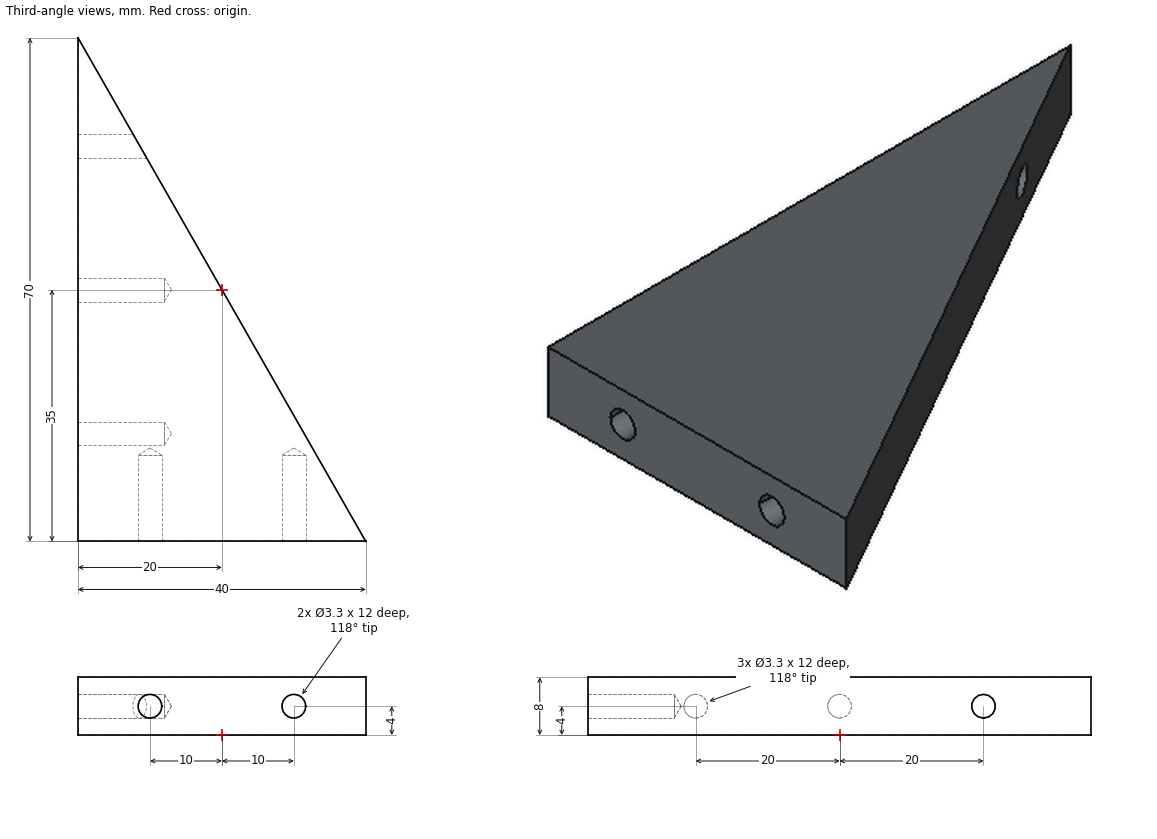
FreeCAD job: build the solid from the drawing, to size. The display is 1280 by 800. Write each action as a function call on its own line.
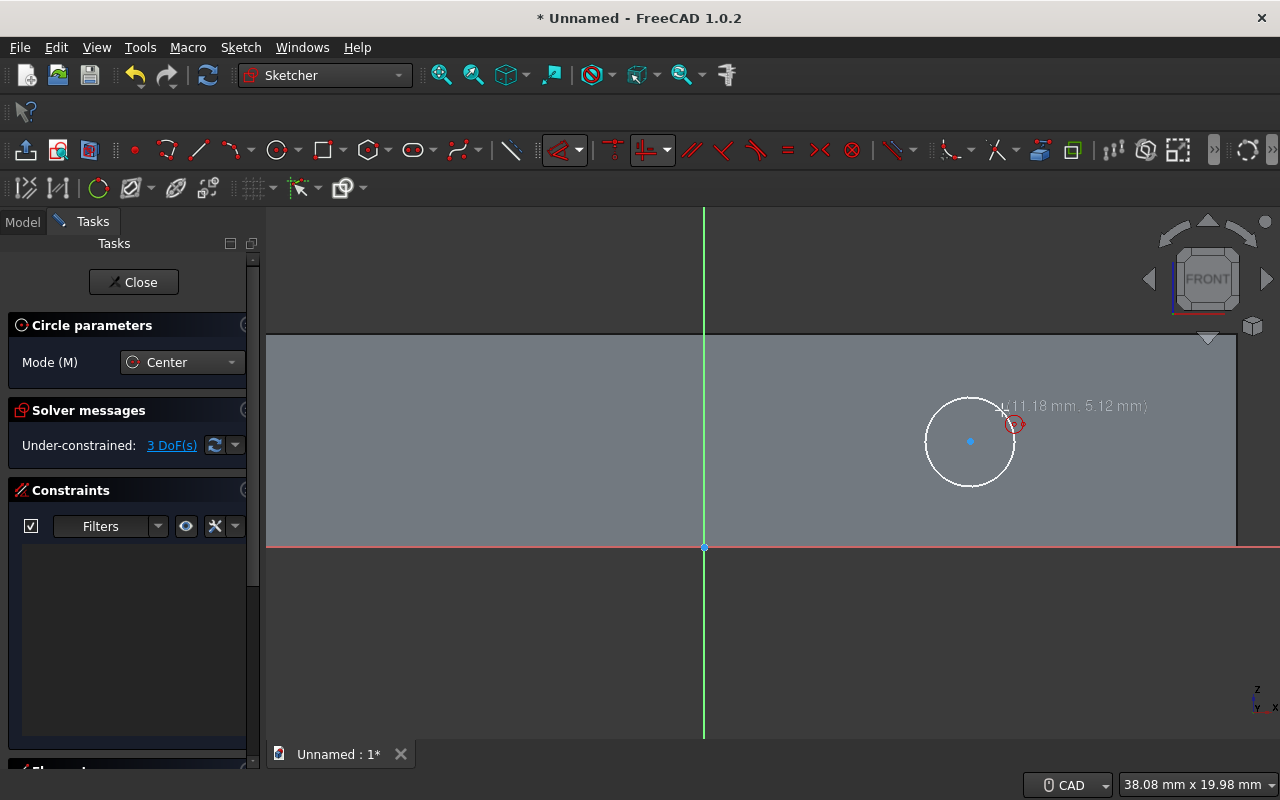
click(438, 441)
click(469, 410)
key(Escape)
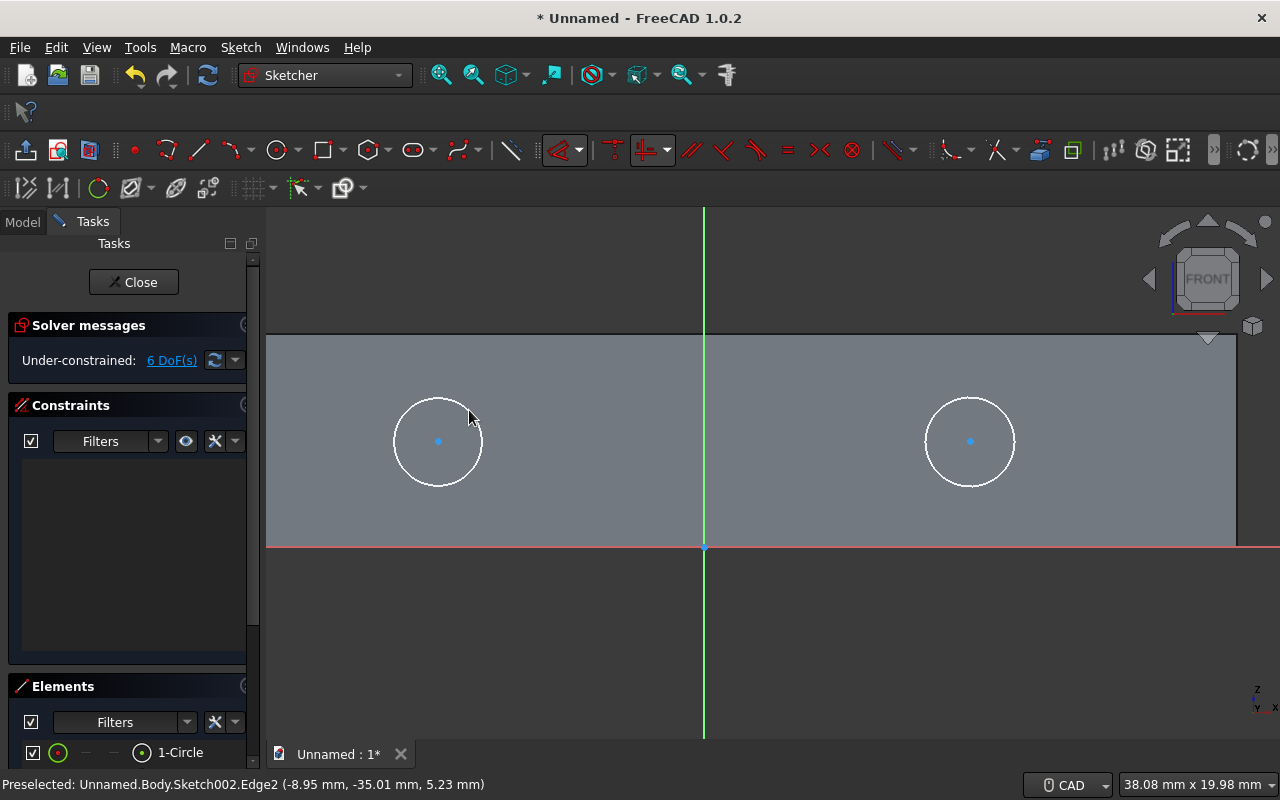
click(1001, 410)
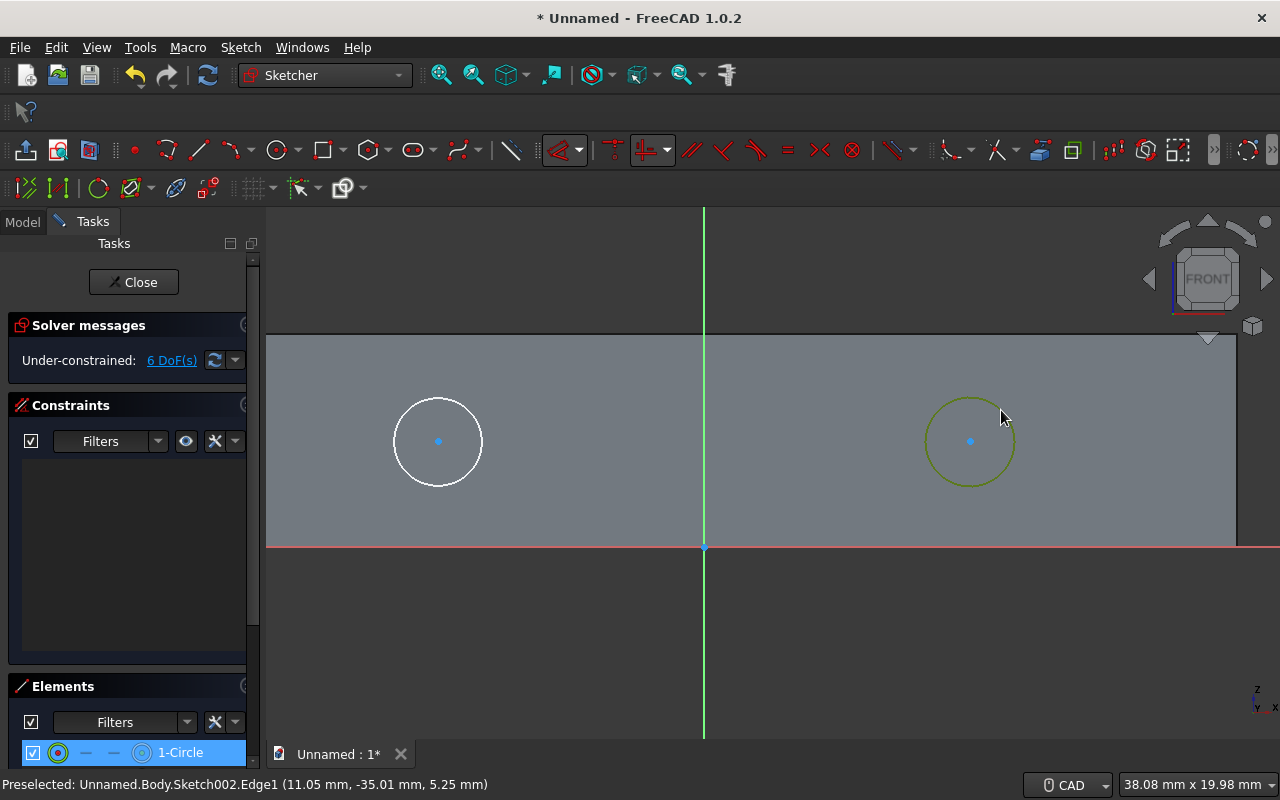
click(469, 411)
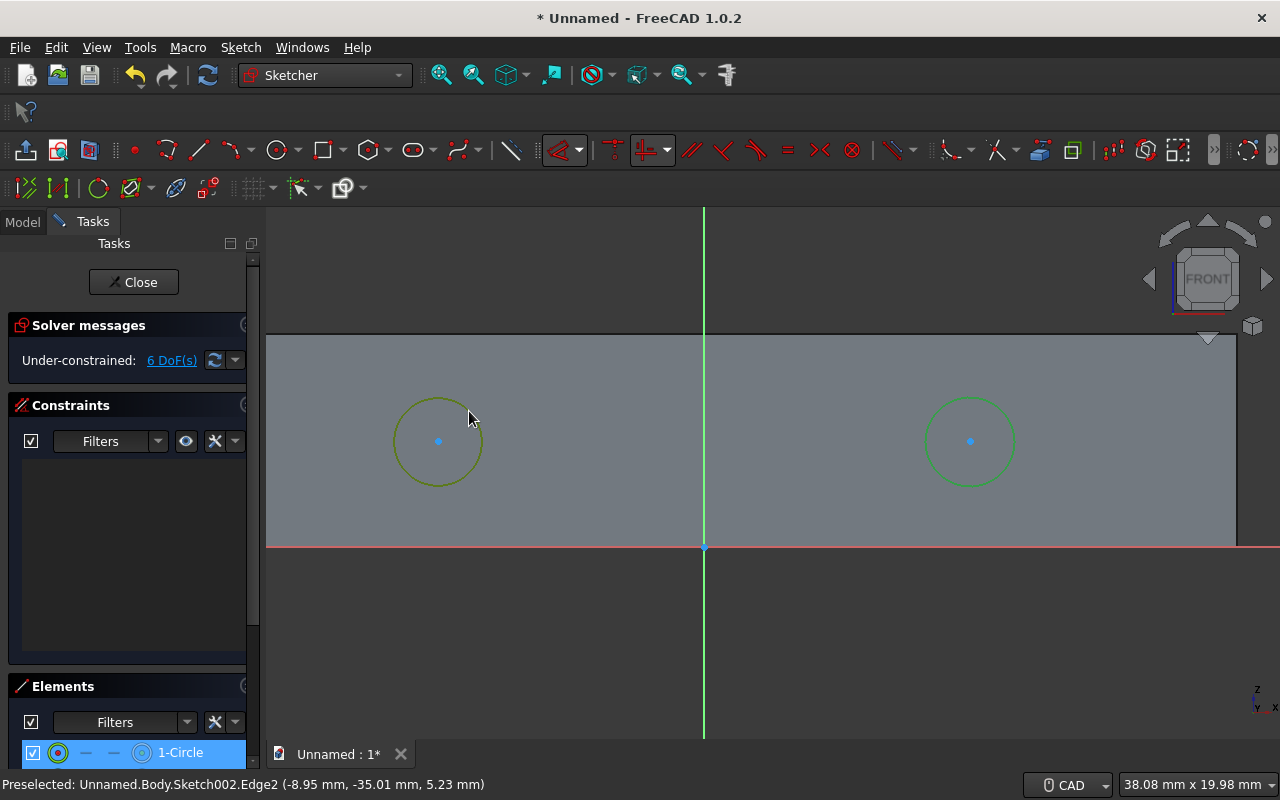
key(e)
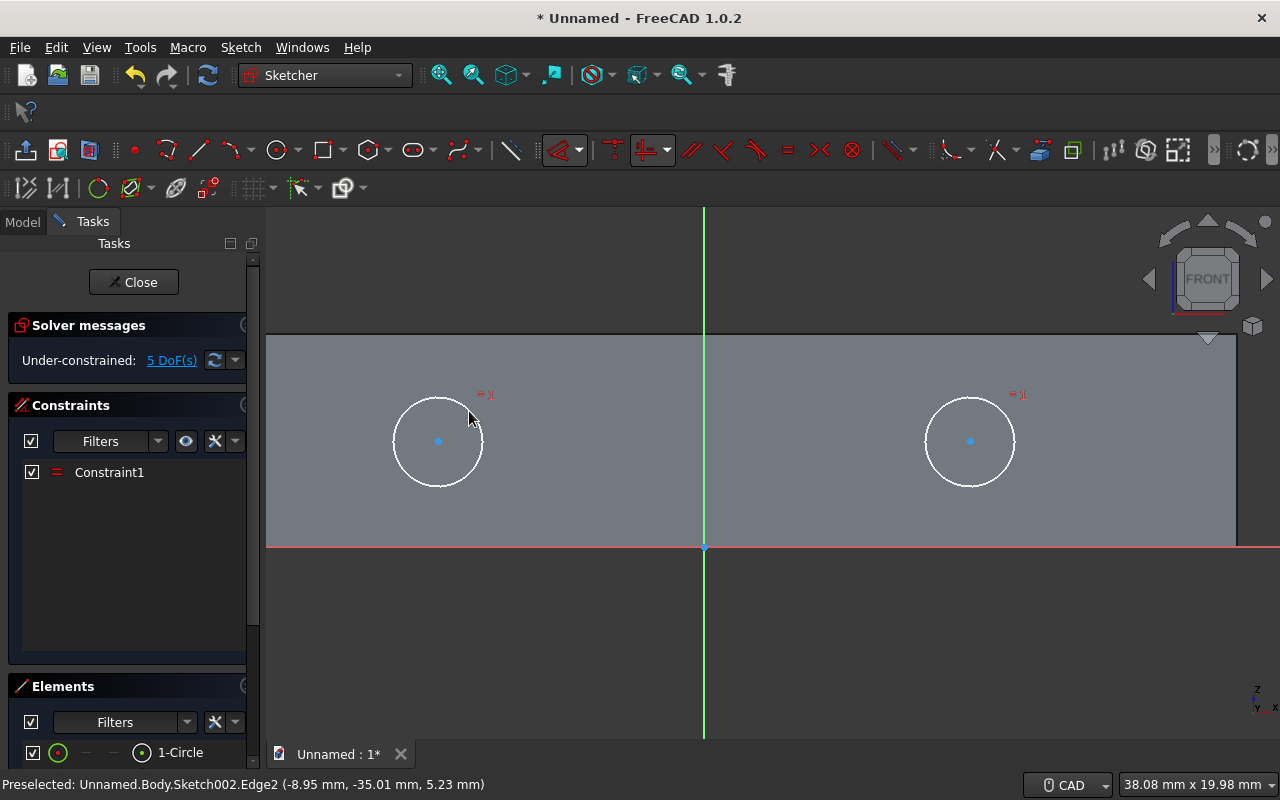
click(970, 442)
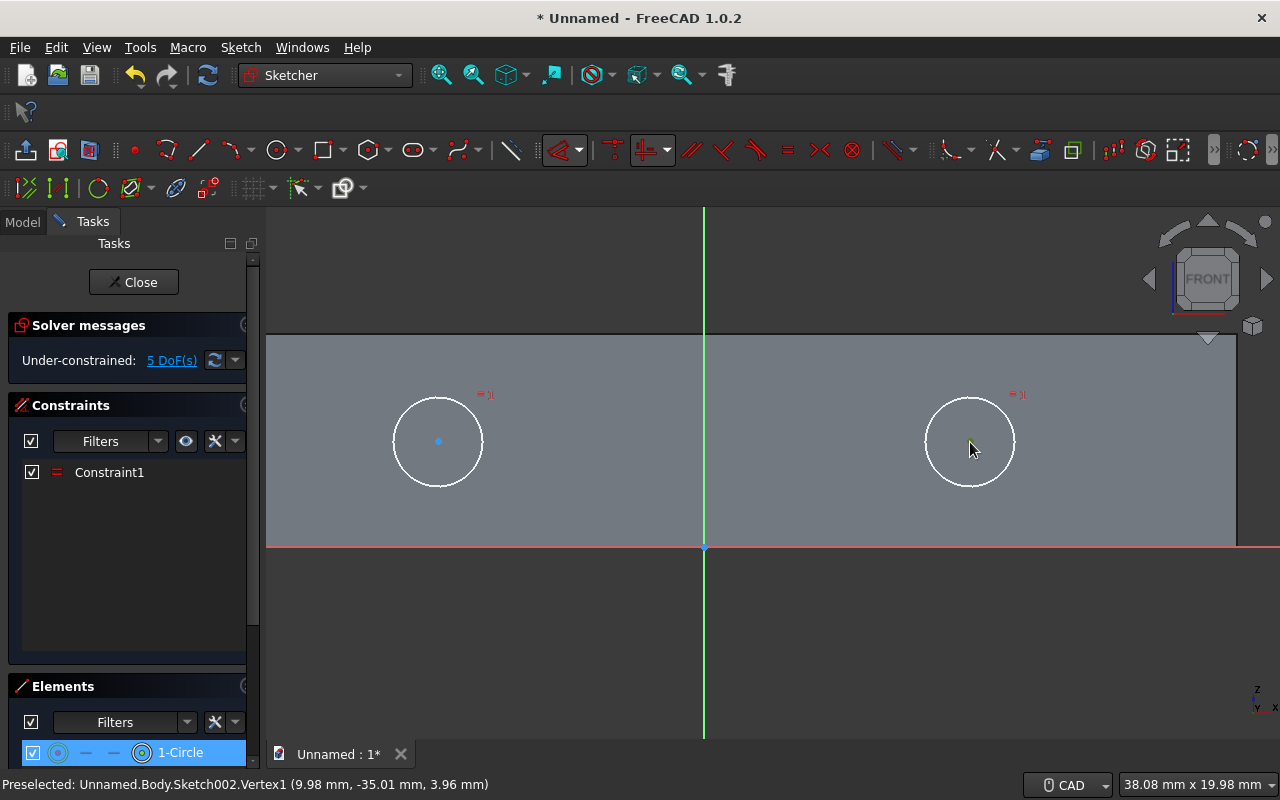
click(438, 442)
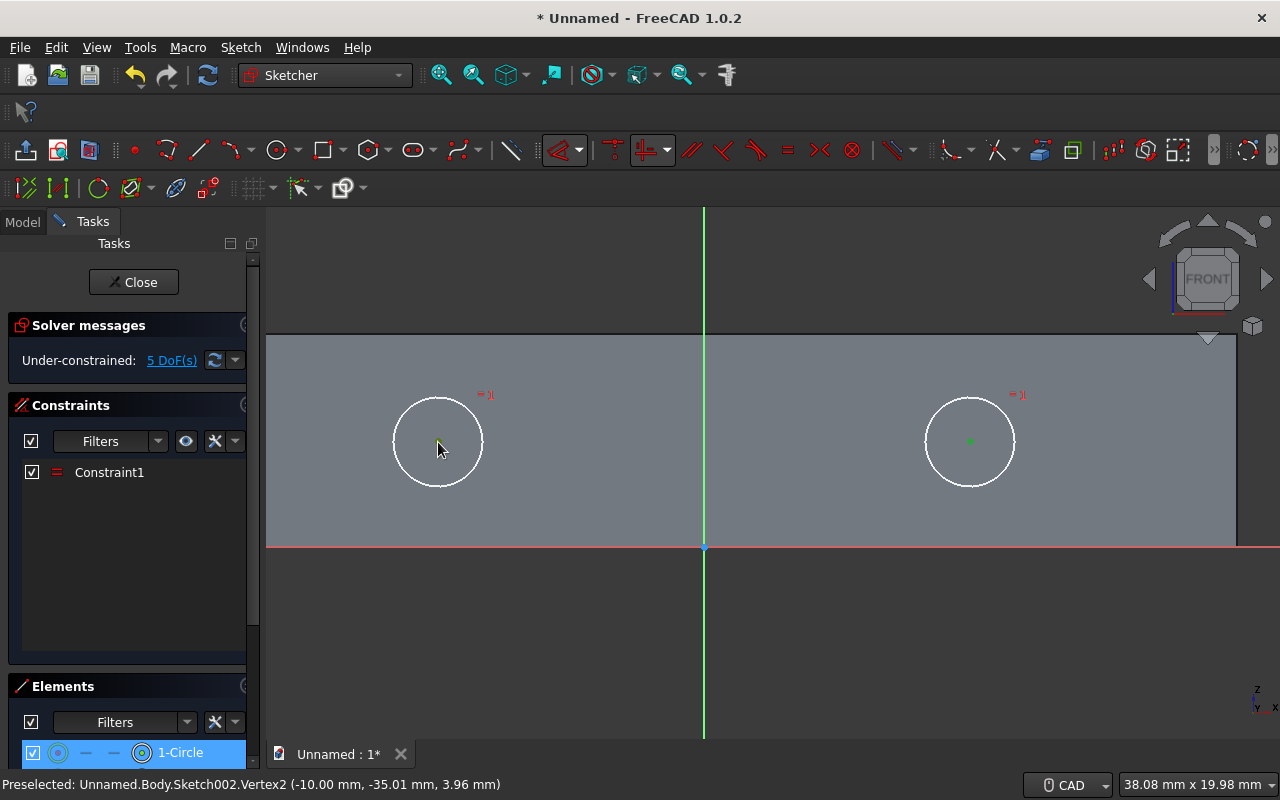
click(670, 150)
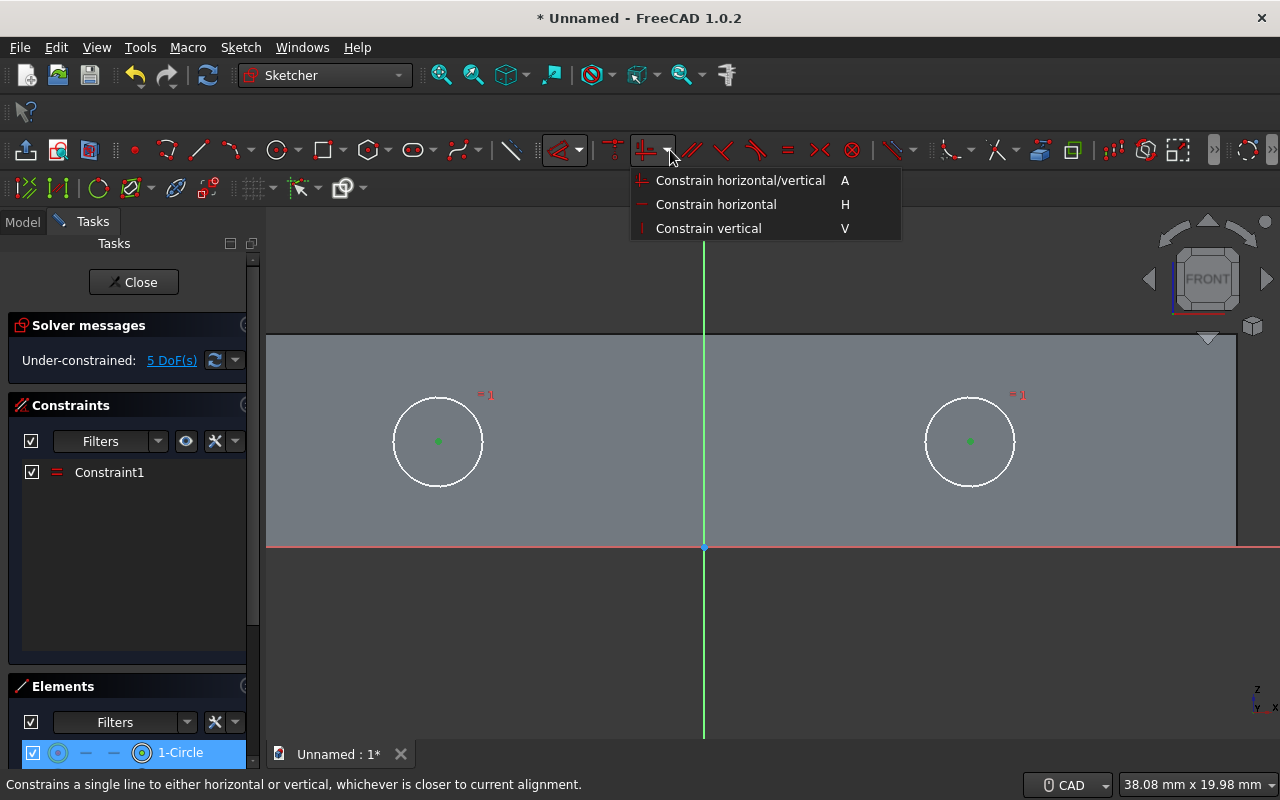
click(766, 204)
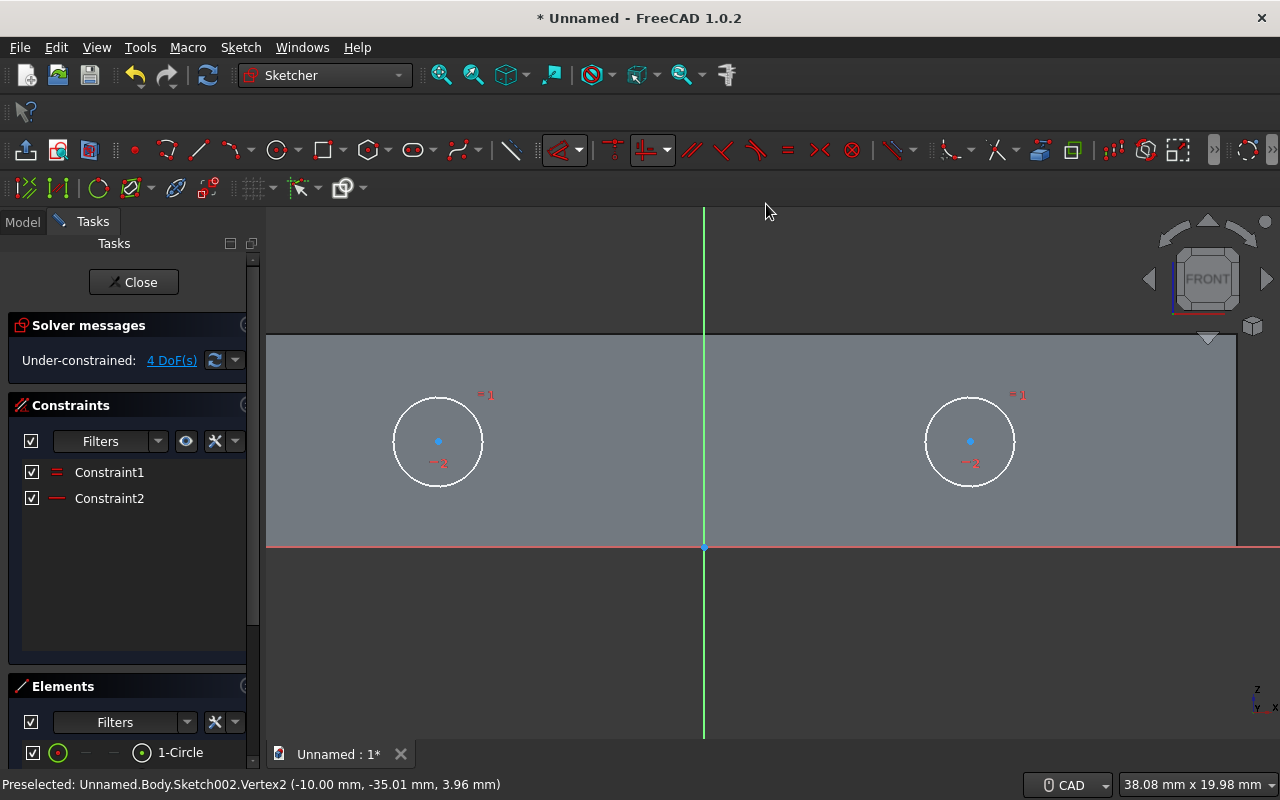
click(1001, 410)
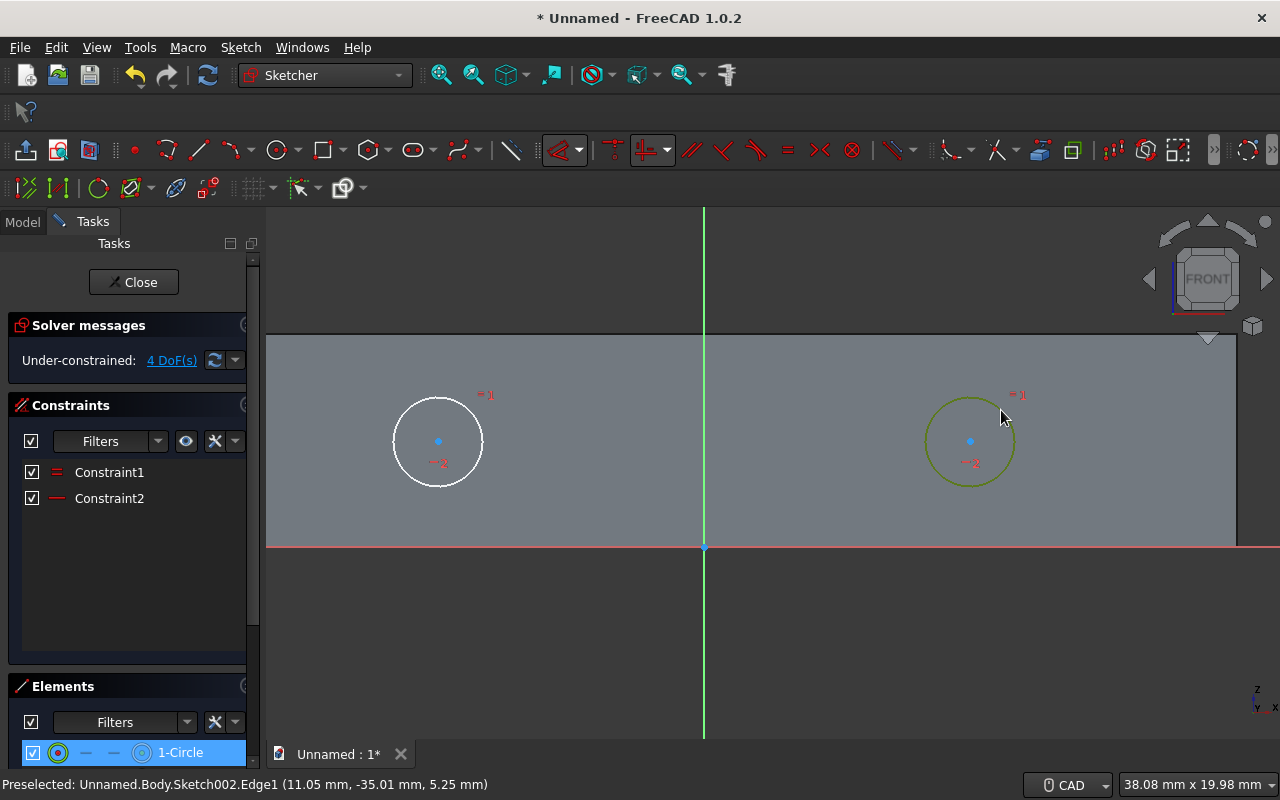
click(582, 150)